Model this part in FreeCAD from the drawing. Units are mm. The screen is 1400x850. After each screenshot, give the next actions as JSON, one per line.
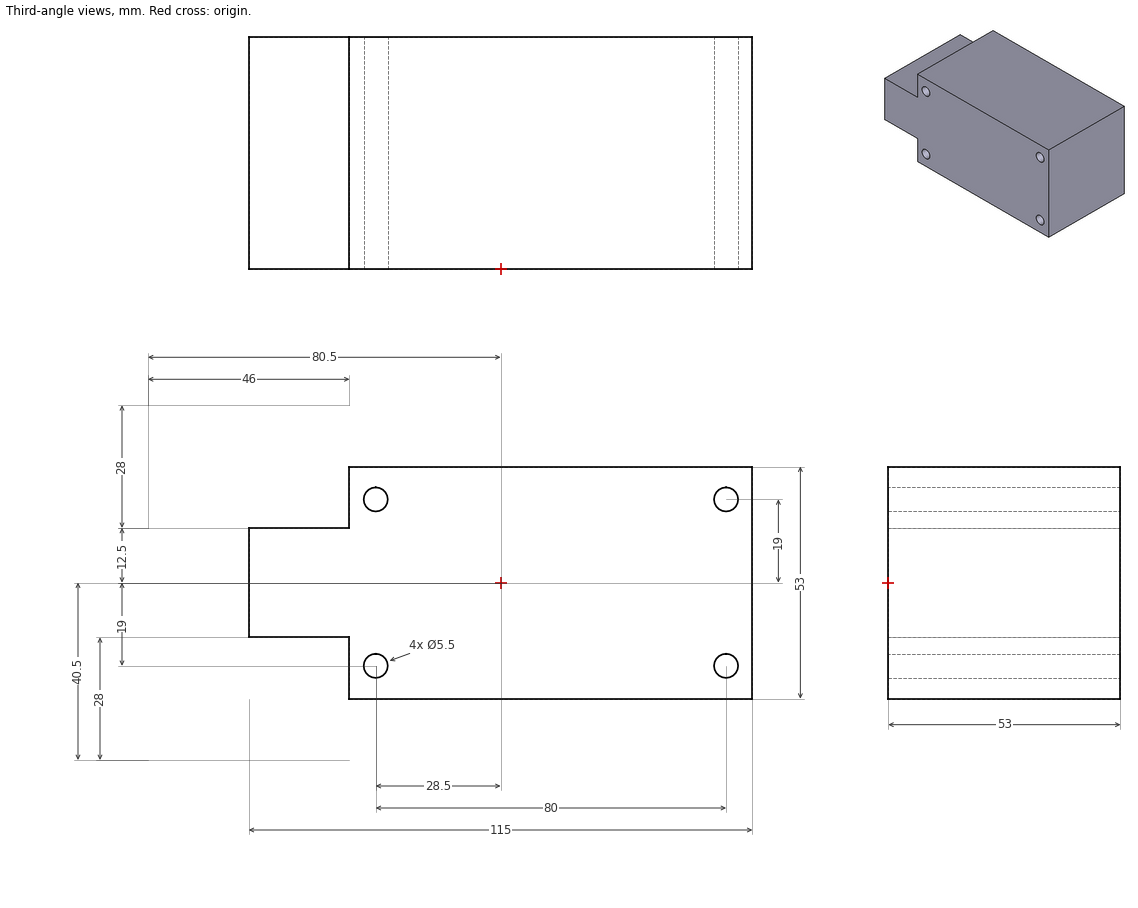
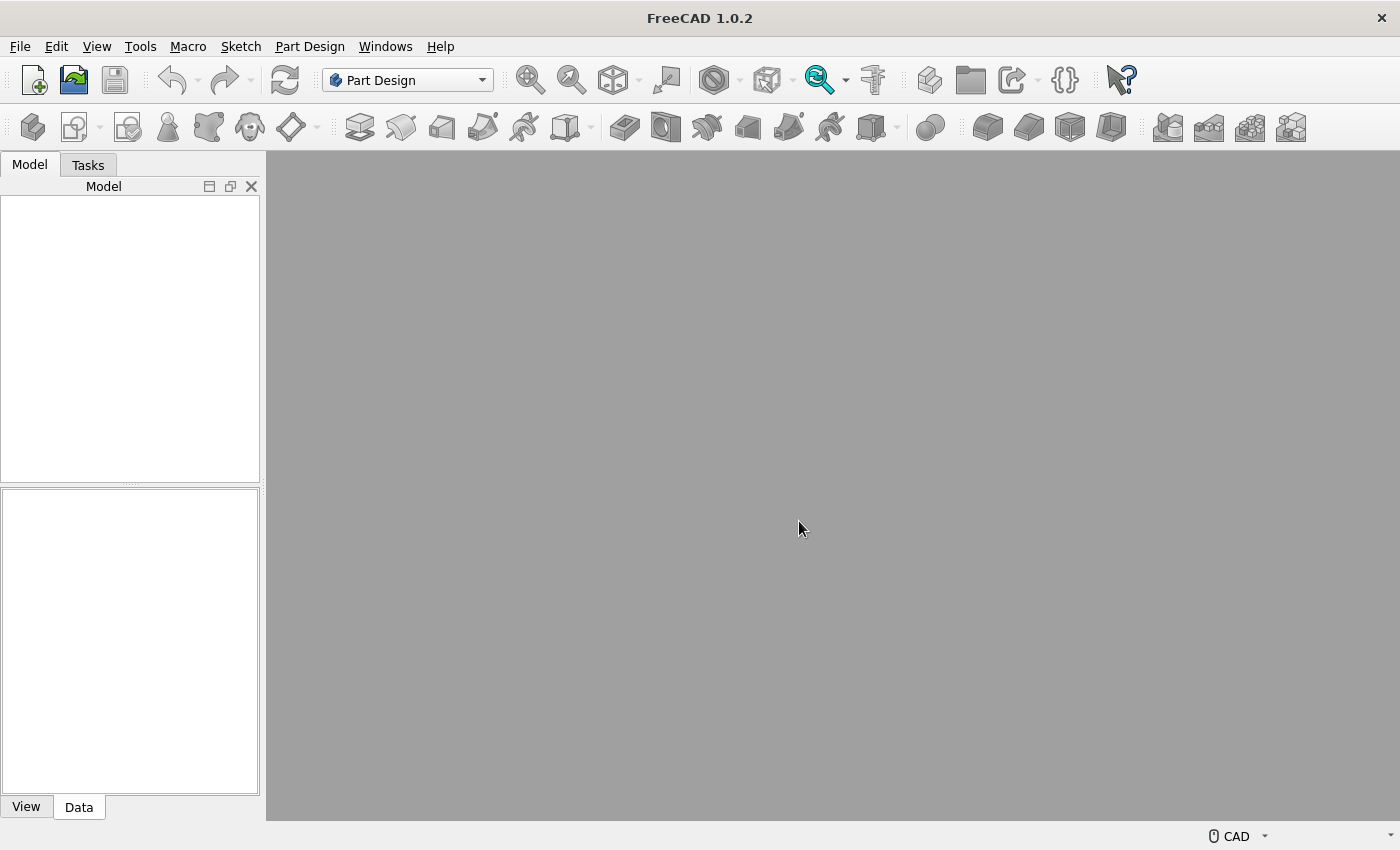
{"action": "left_click", "coordinate": [33, 80]}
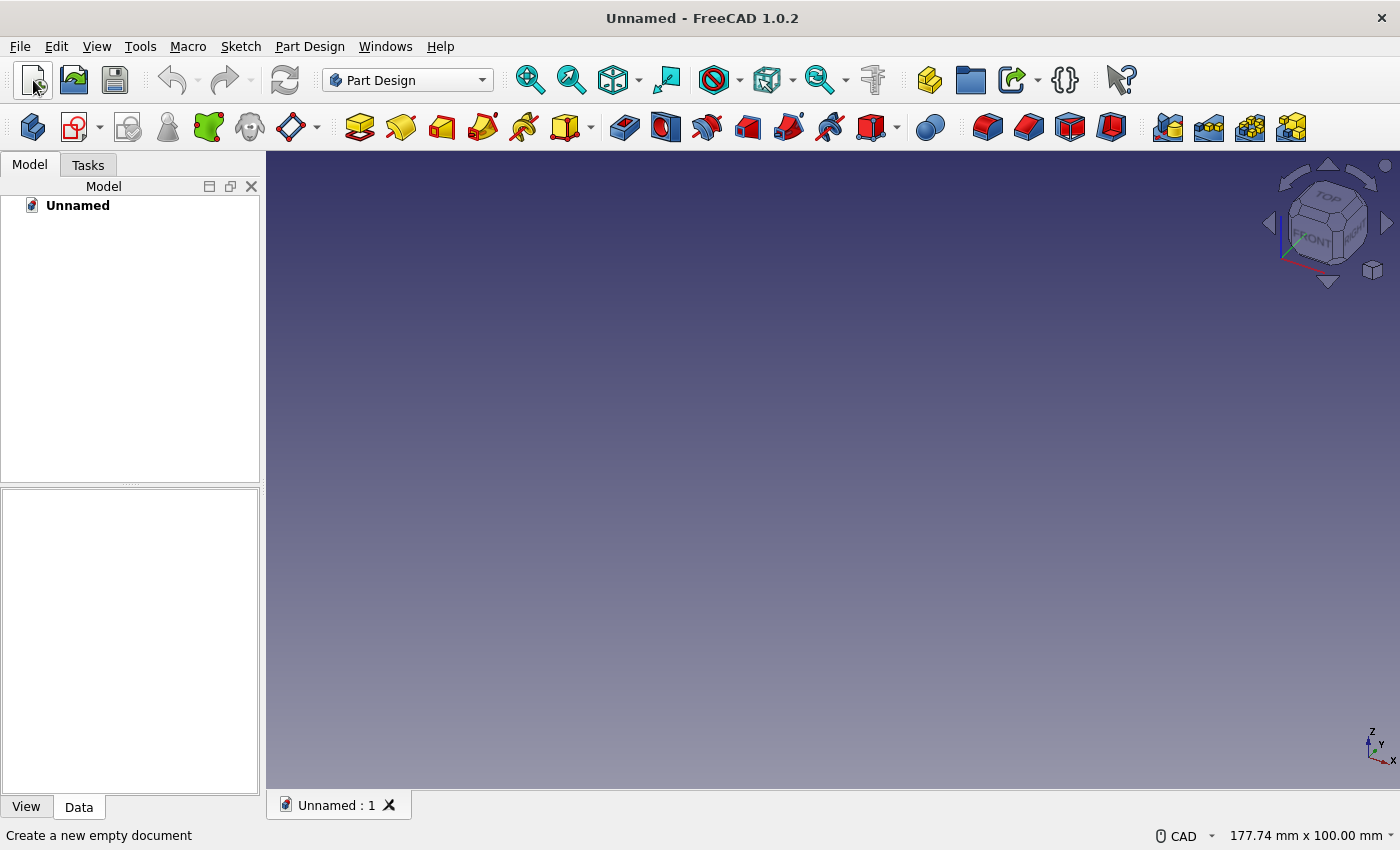
{"action": "left_click", "coordinate": [74, 128]}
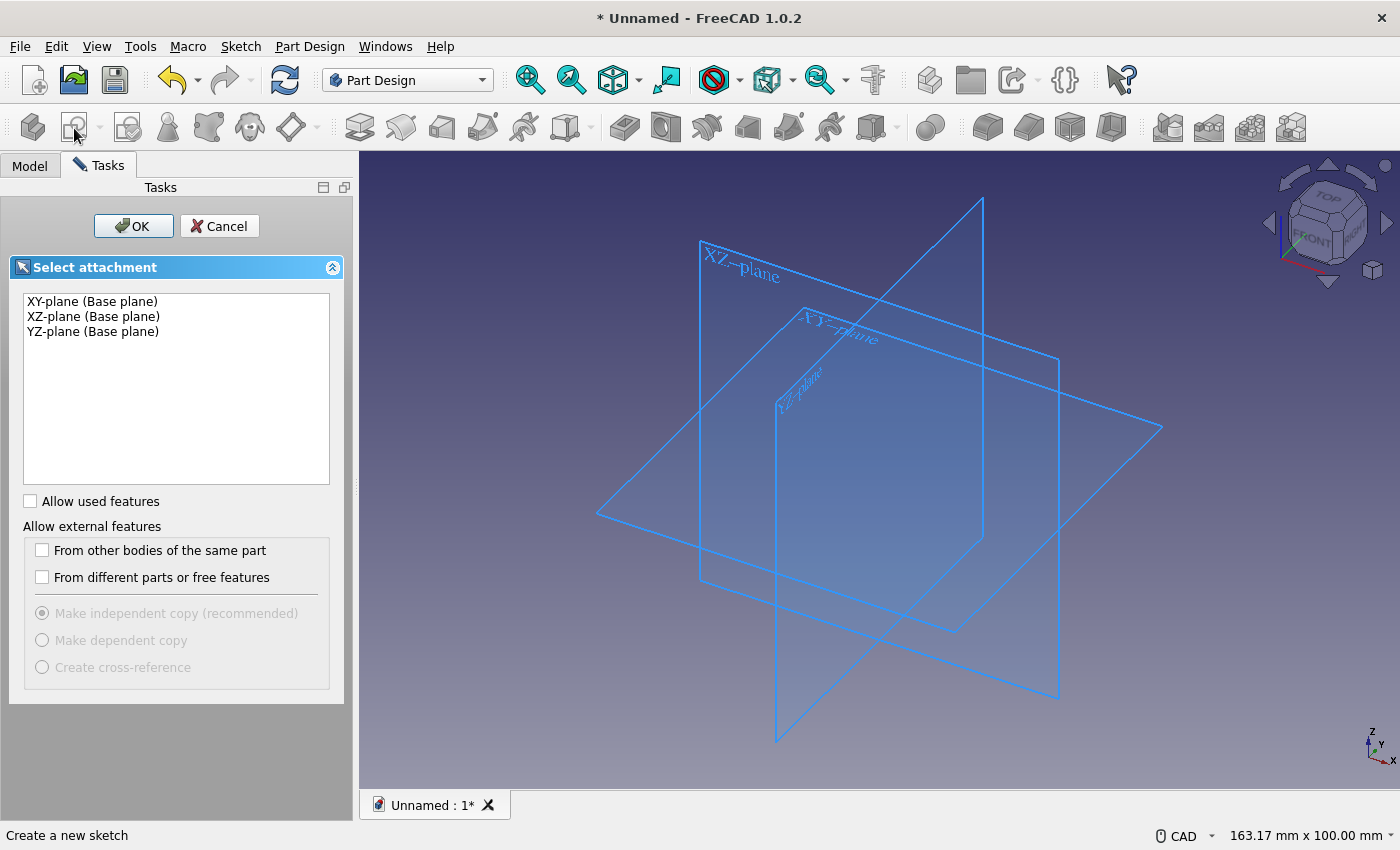
{"action": "left_click", "coordinate": [84, 316]}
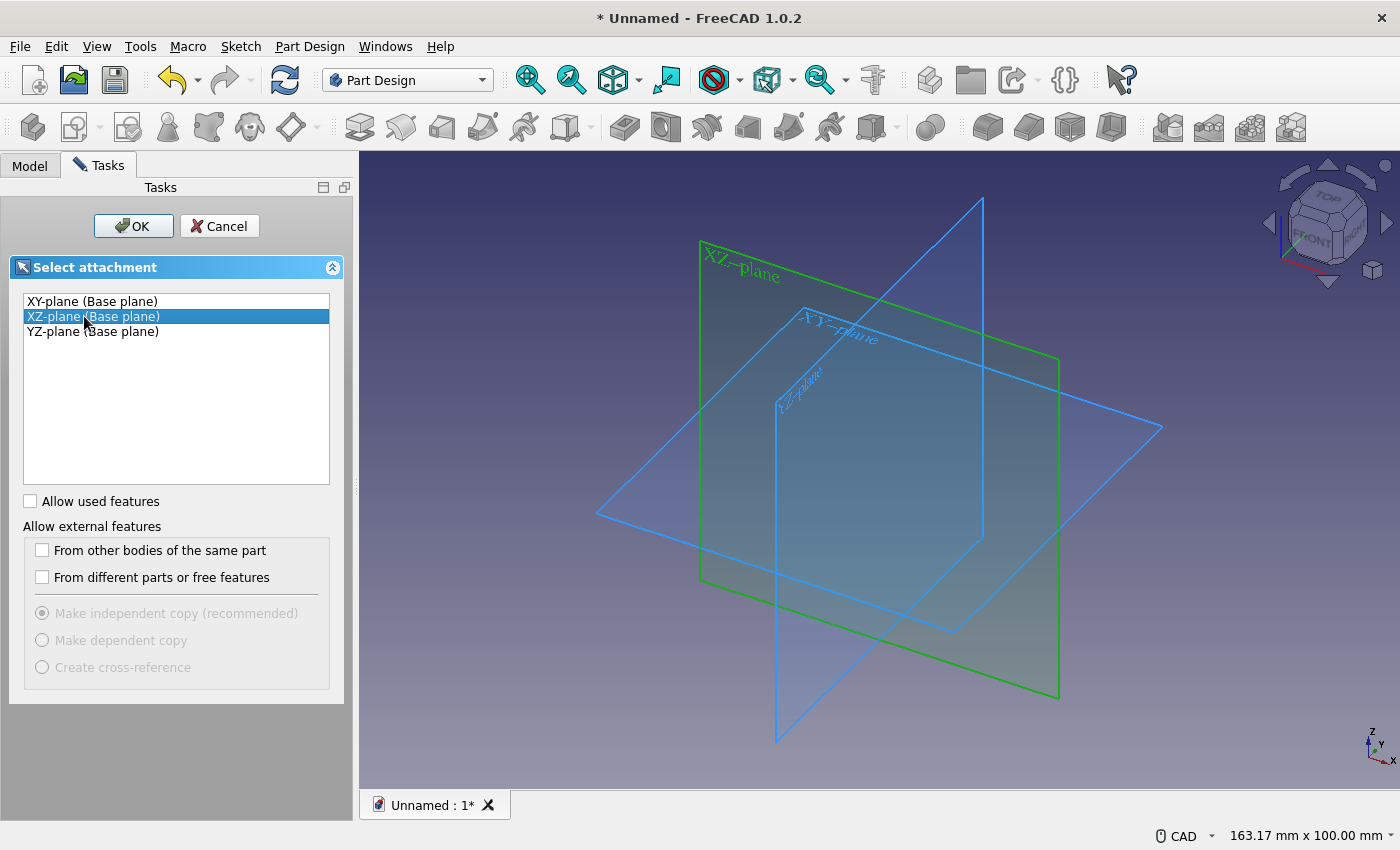
{"action": "left_click", "coordinate": [134, 226]}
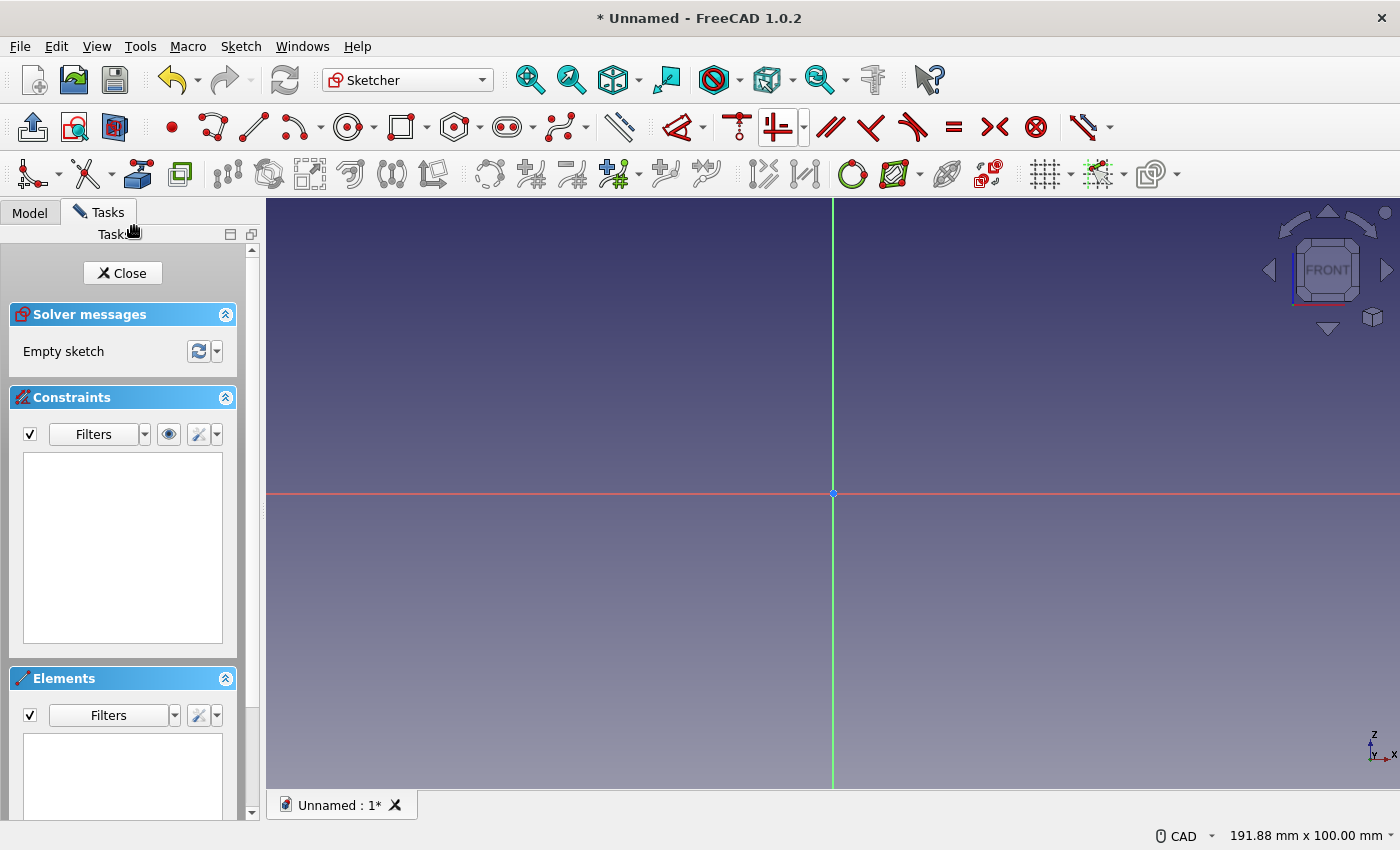
{"action": "left_click", "coordinate": [426, 128]}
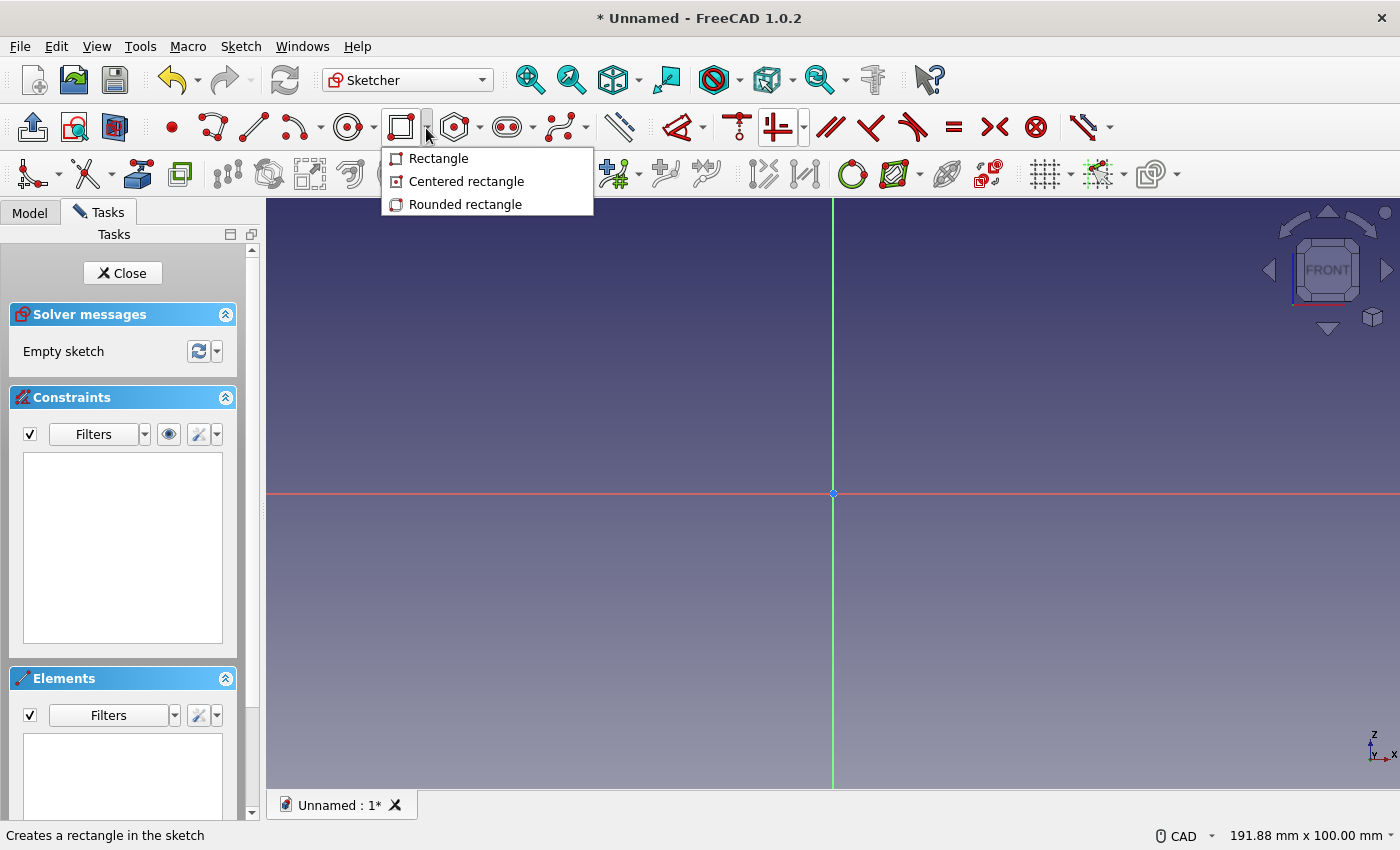
{"action": "left_click", "coordinate": [488, 182]}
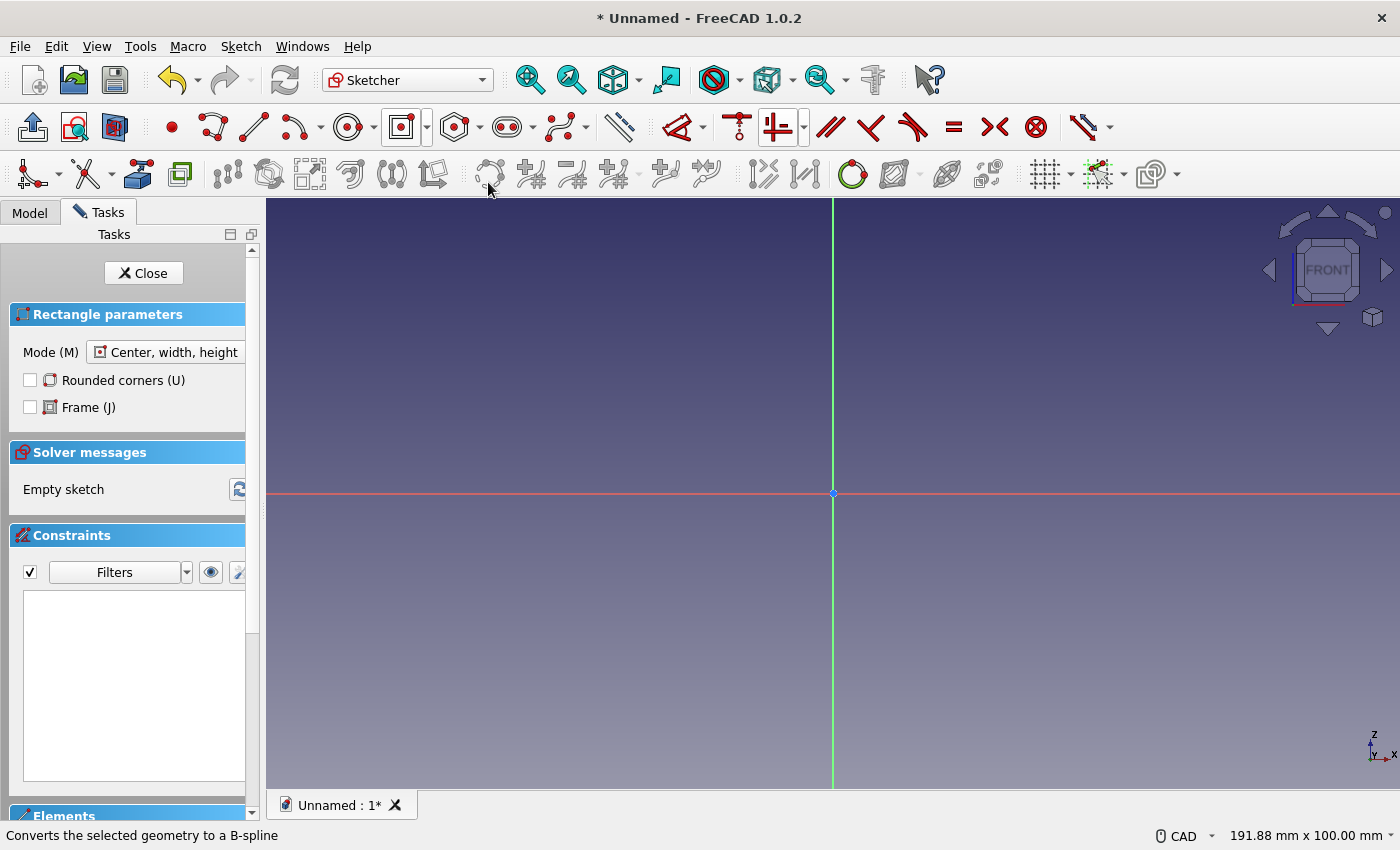
{"action": "left_click", "coordinate": [833, 494]}
{"action": "mouse_move", "coordinate": [1173, 337]}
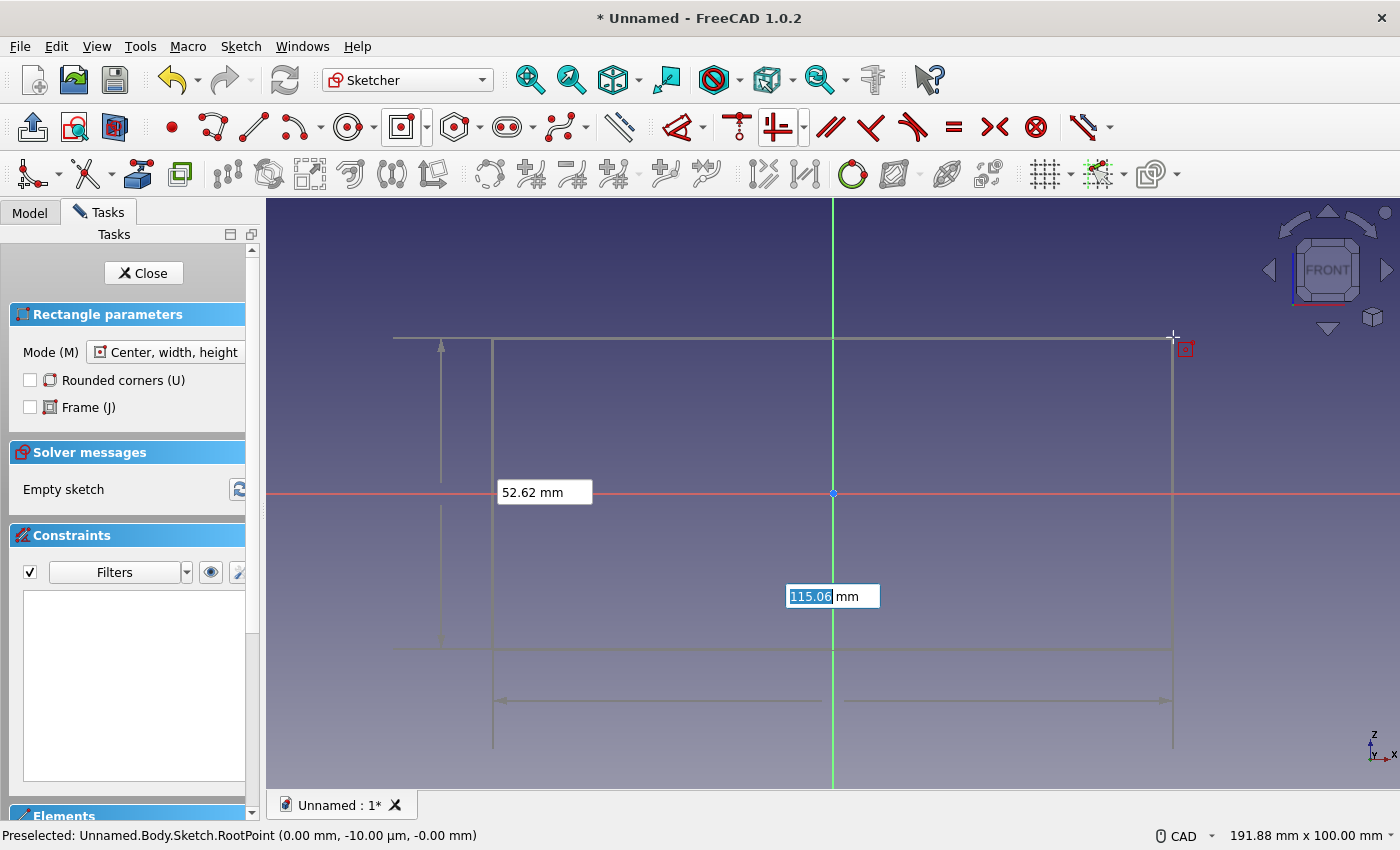
{"action": "type", "text": "115"}
{"action": "key", "text": "Tab"}
{"action": "type", "text": "53"}
{"action": "key", "text": "Return"}
{"action": "key", "text": "Escape"}